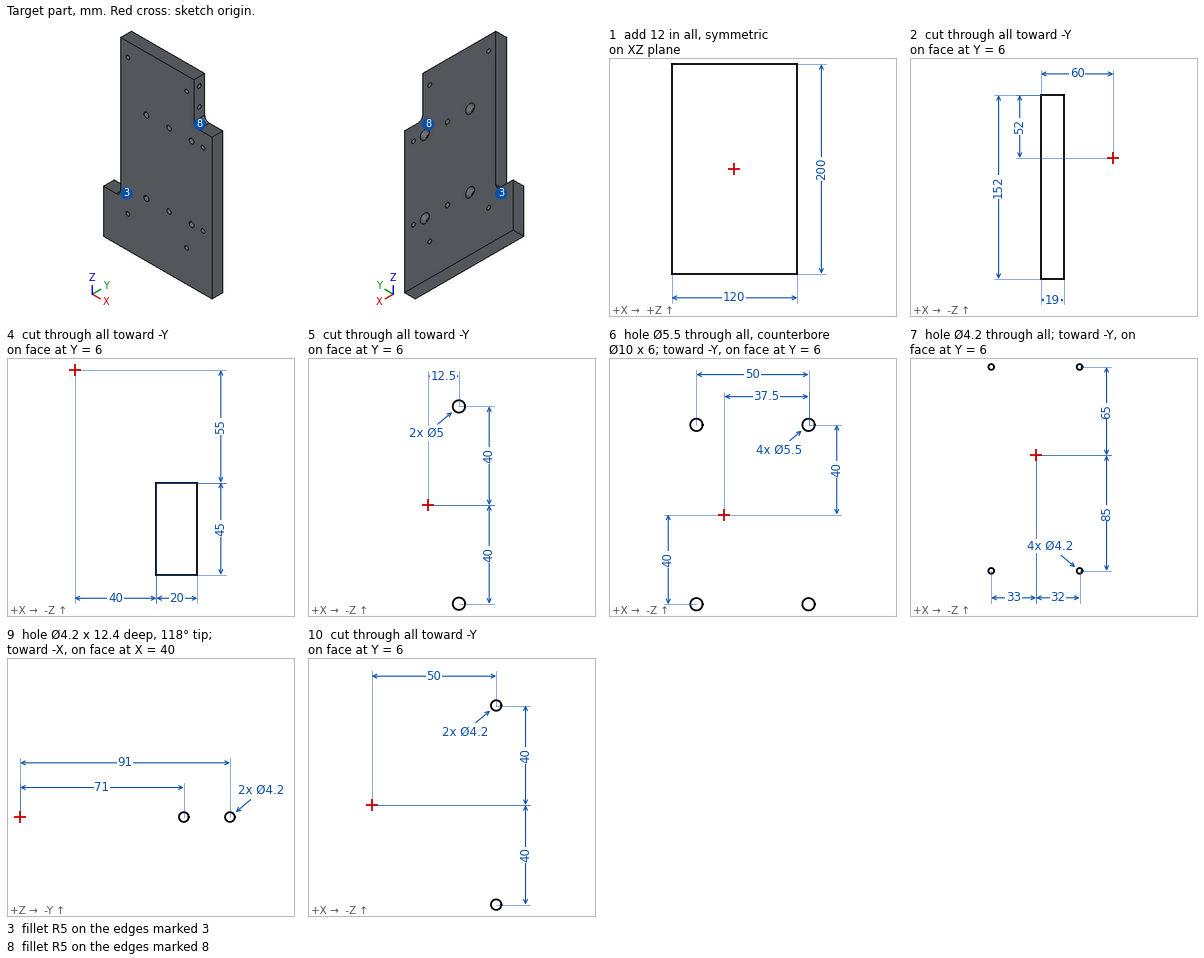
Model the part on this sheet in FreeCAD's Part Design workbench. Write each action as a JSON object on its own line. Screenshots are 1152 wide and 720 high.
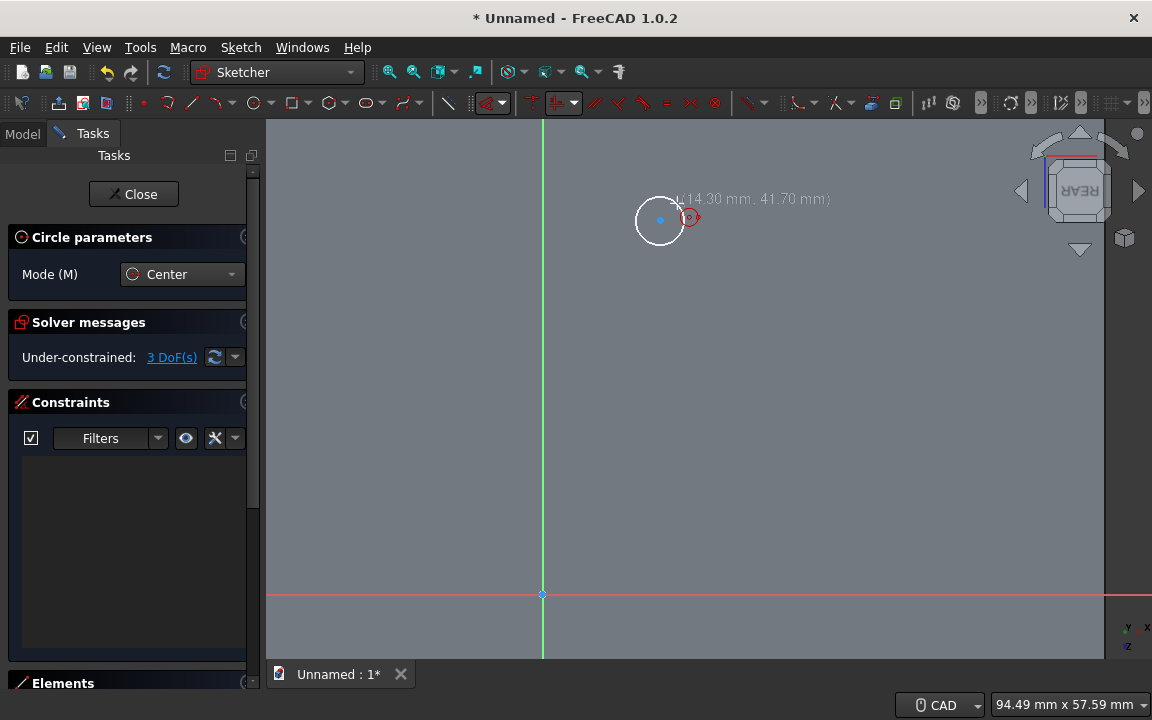
{"action": "scroll", "coordinate": [663, 221], "scroll_direction": "down", "scroll_amount": 4}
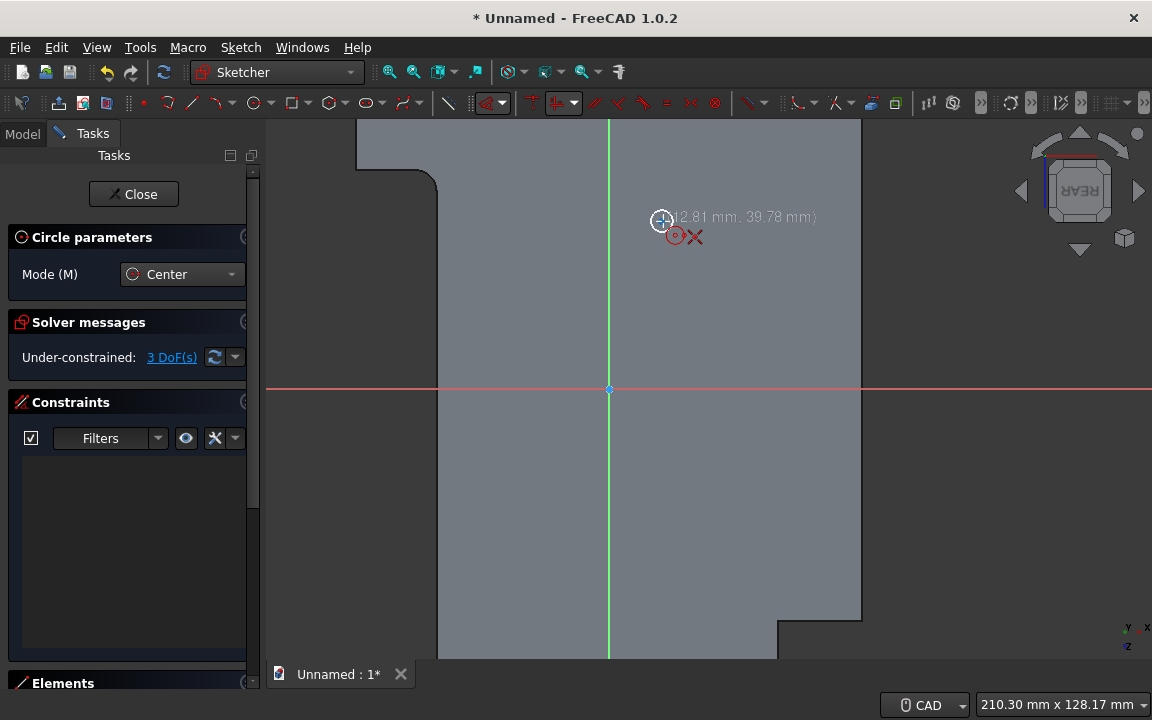
{"action": "scroll", "coordinate": [662, 558], "scroll_direction": "up", "scroll_amount": 4}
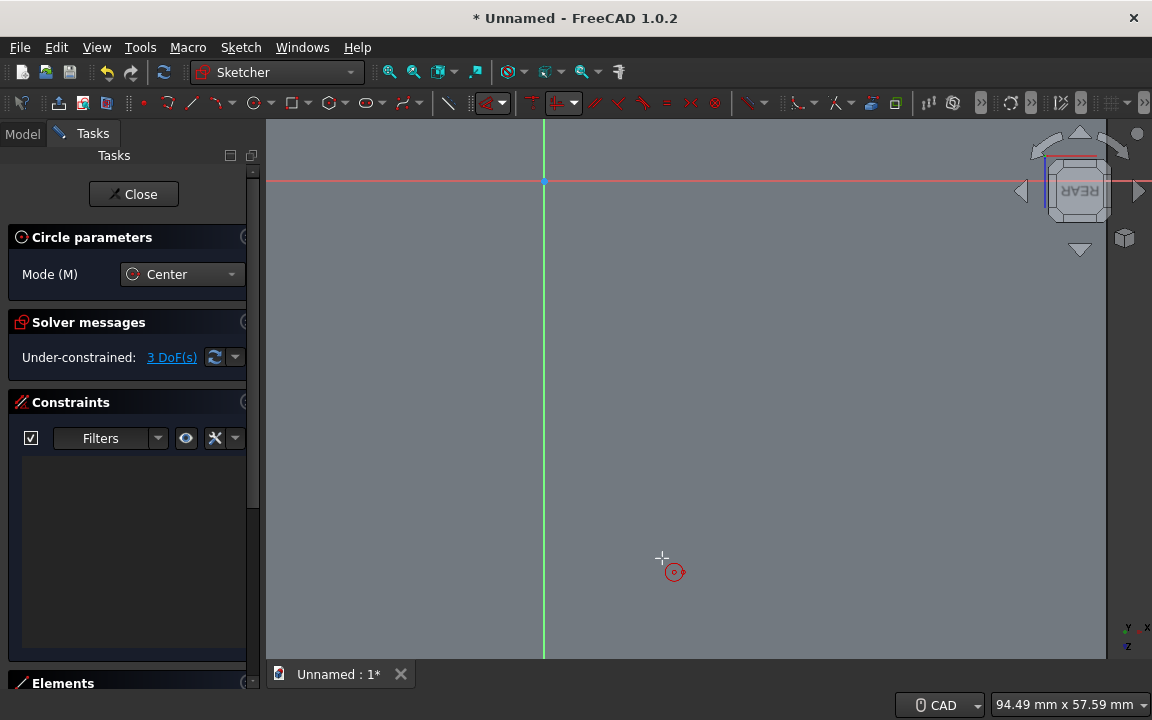
{"action": "left_click", "coordinate": [661, 556]}
{"action": "left_click", "coordinate": [678, 540]}
{"action": "key", "text": "Escape"}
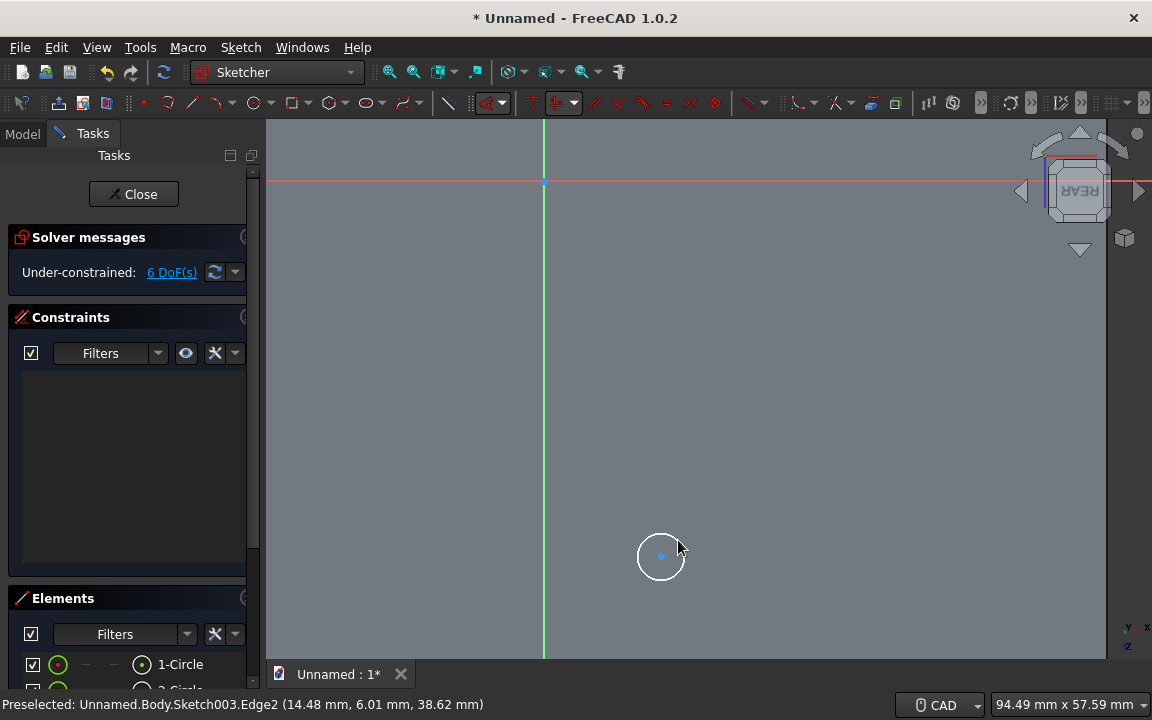
{"action": "scroll", "coordinate": [662, 559], "scroll_direction": "down", "scroll_amount": 4}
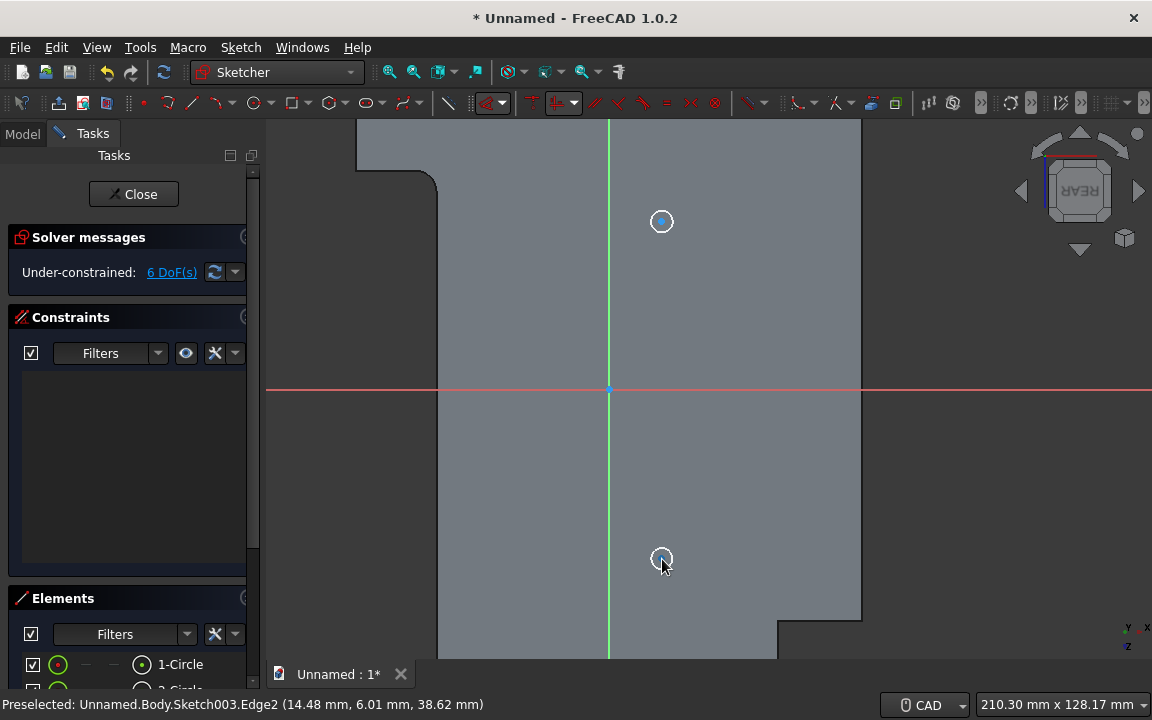
{"action": "scroll", "coordinate": [670, 214], "scroll_direction": "up", "scroll_amount": 2}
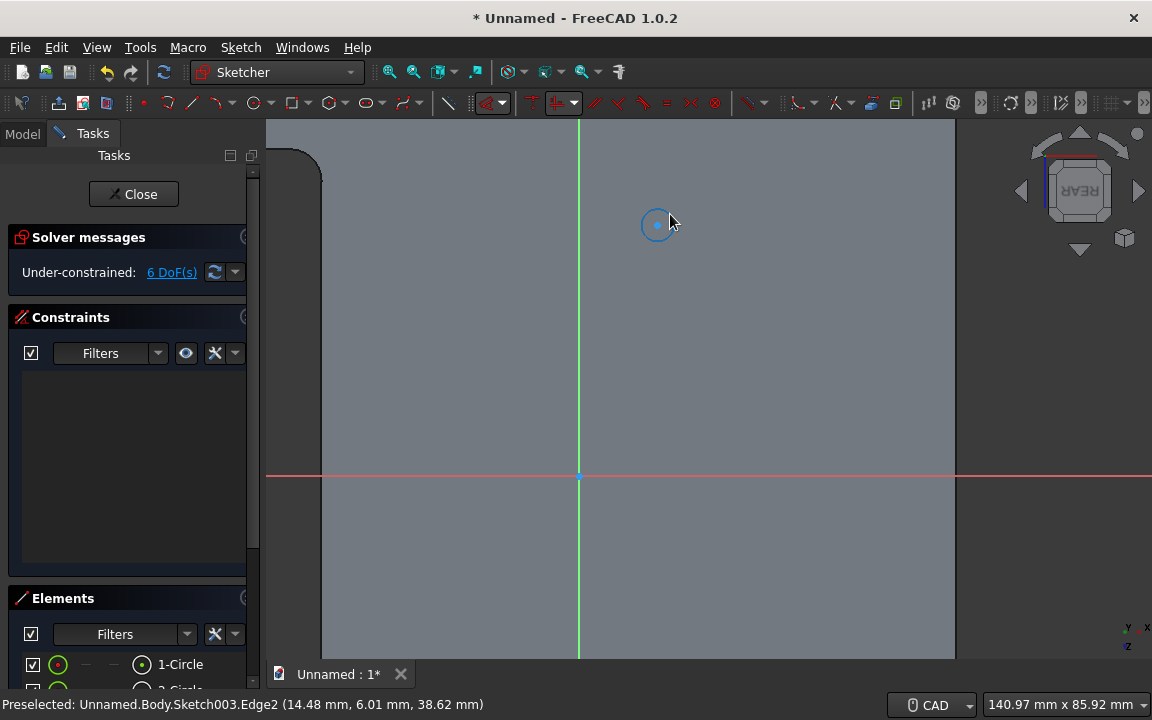
{"action": "left_click", "coordinate": [669, 214]}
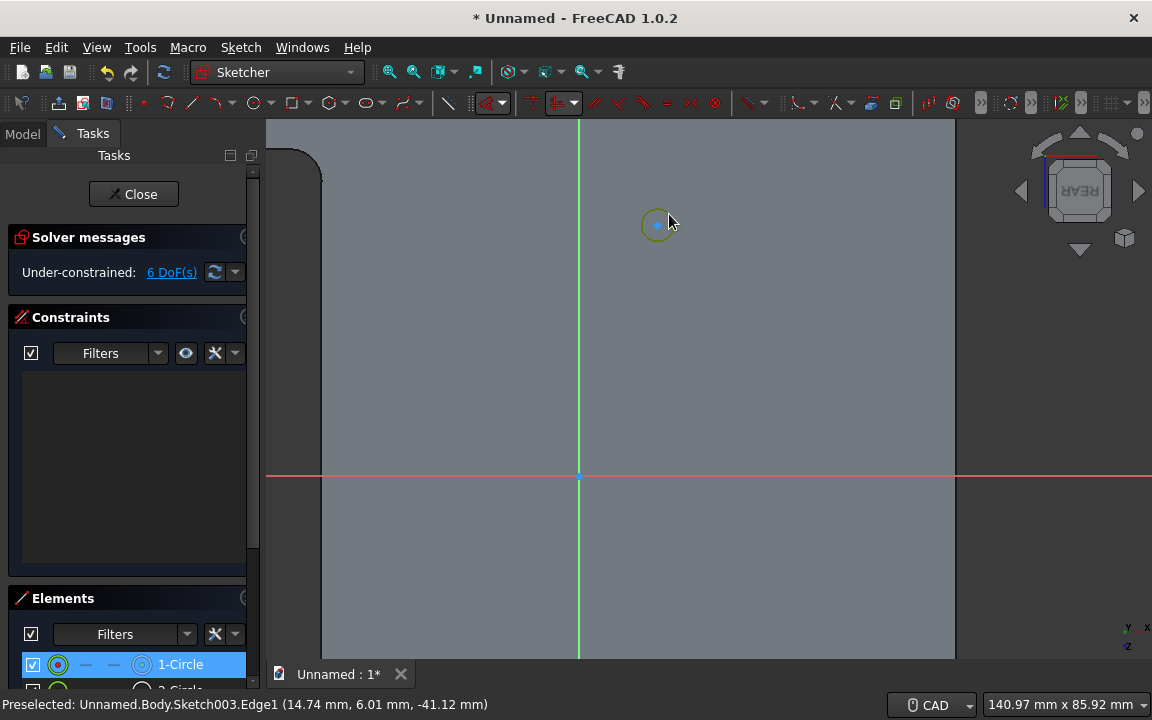
{"action": "scroll", "coordinate": [669, 212], "scroll_direction": "down", "scroll_amount": 2}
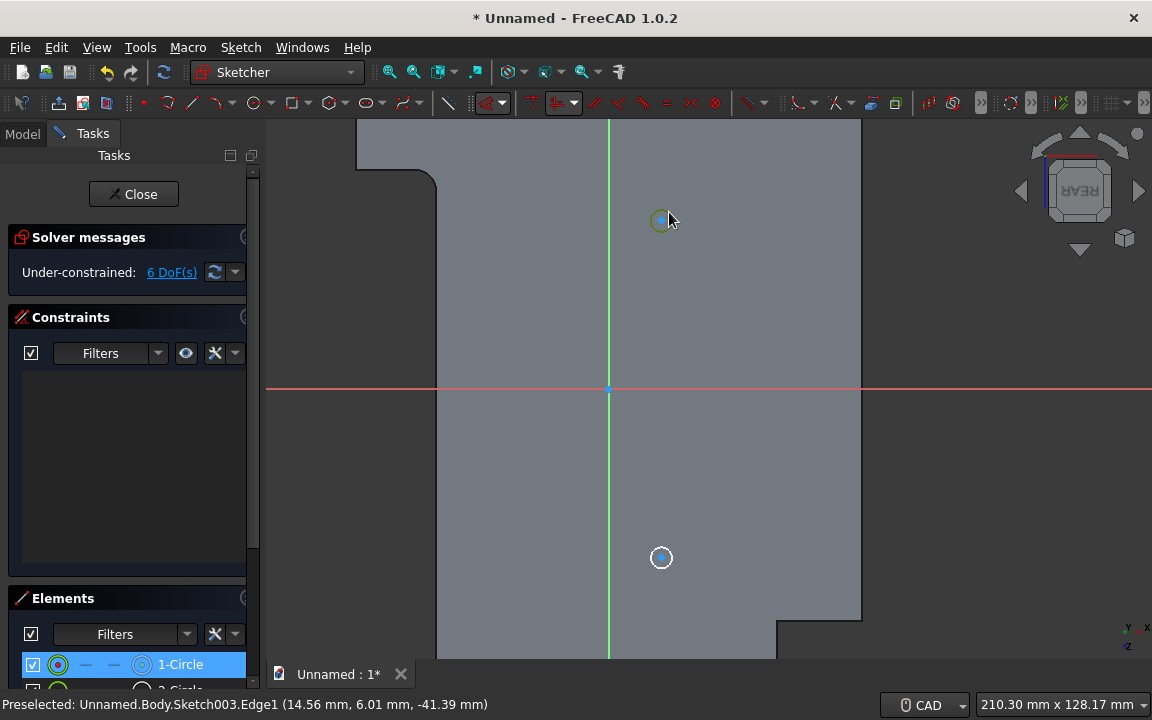
{"action": "scroll", "coordinate": [669, 550], "scroll_direction": "up", "scroll_amount": 2}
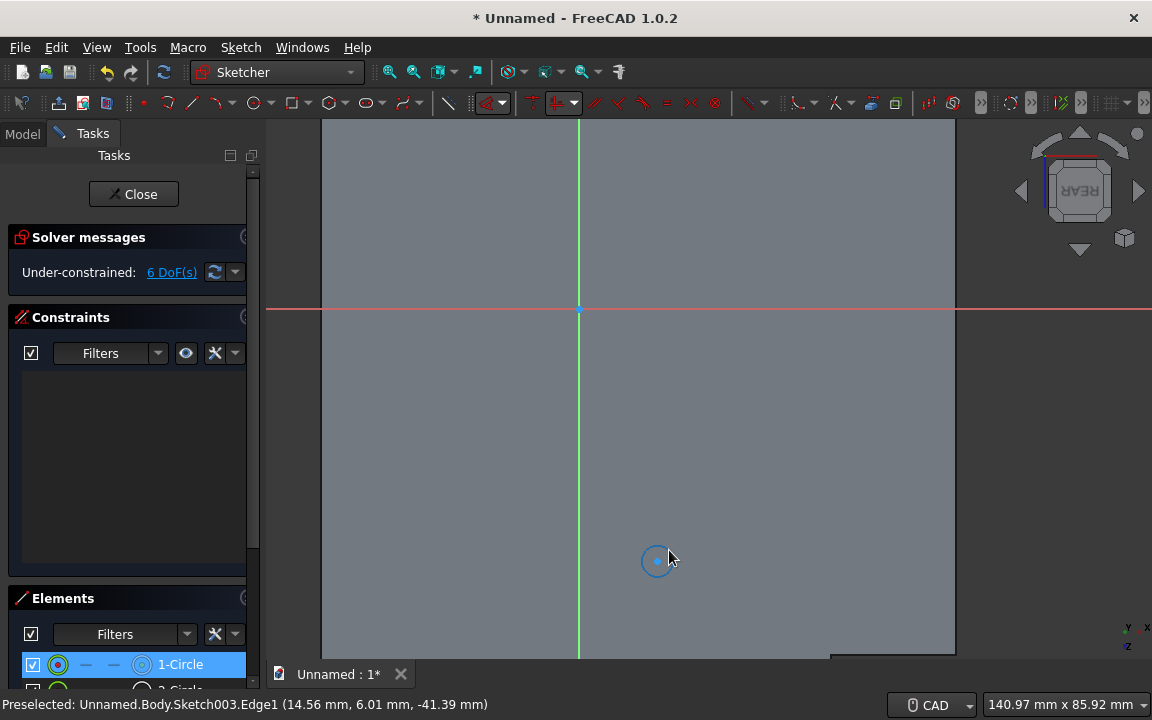
{"action": "left_click", "coordinate": [669, 550]}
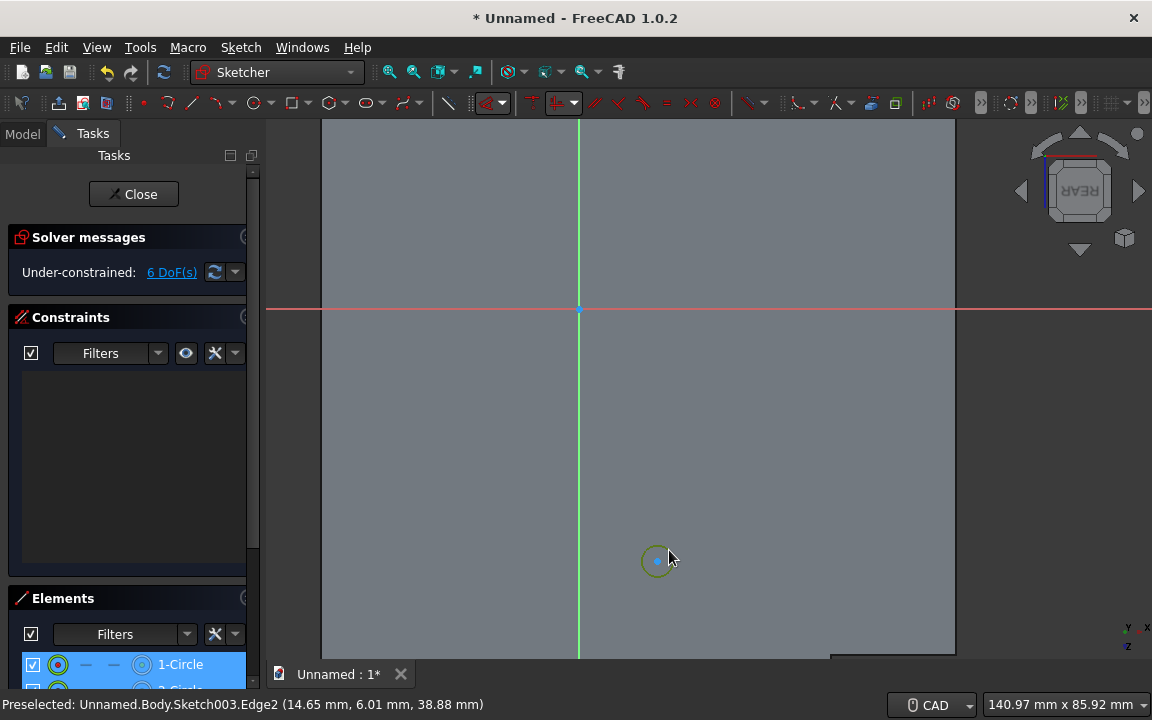
{"action": "left_click", "coordinate": [668, 104]}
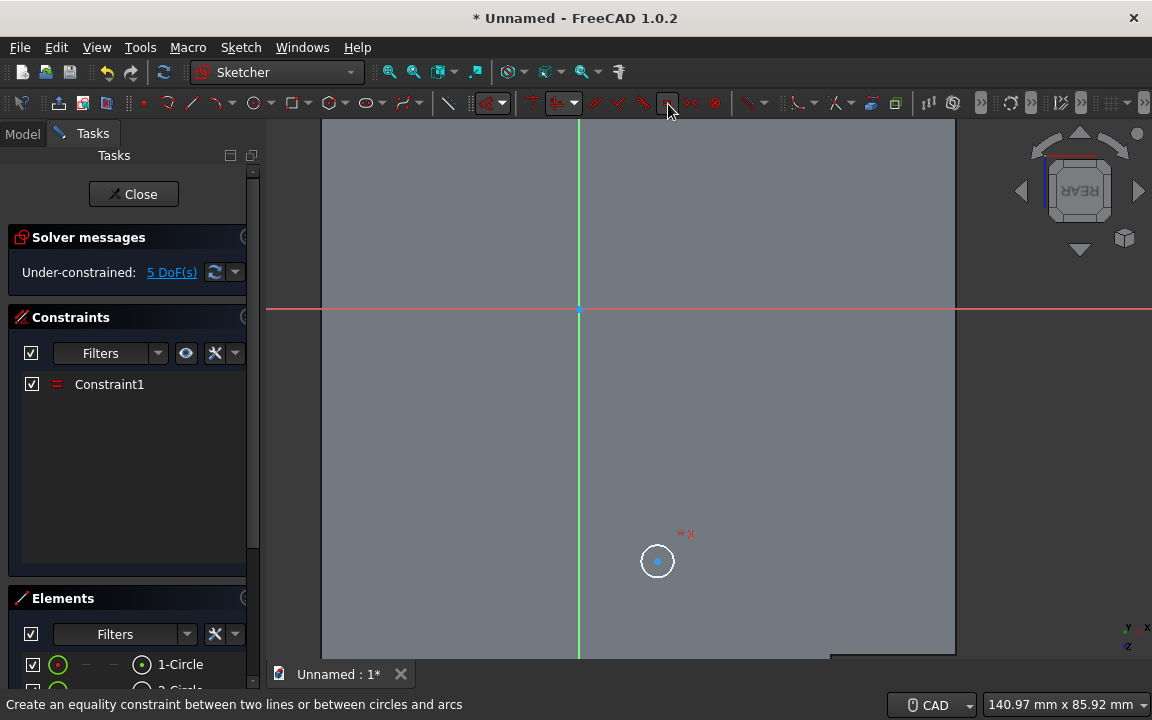
{"action": "scroll", "coordinate": [669, 551], "scroll_direction": "down", "scroll_amount": 2}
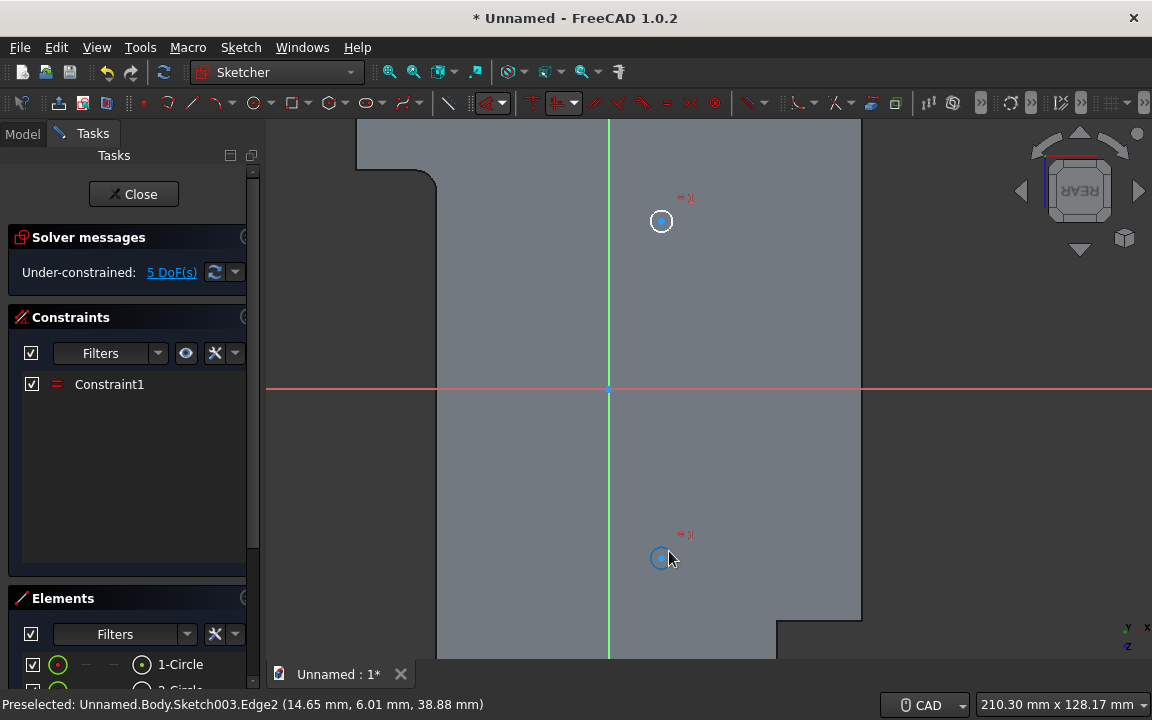
{"action": "left_click", "coordinate": [662, 221]}